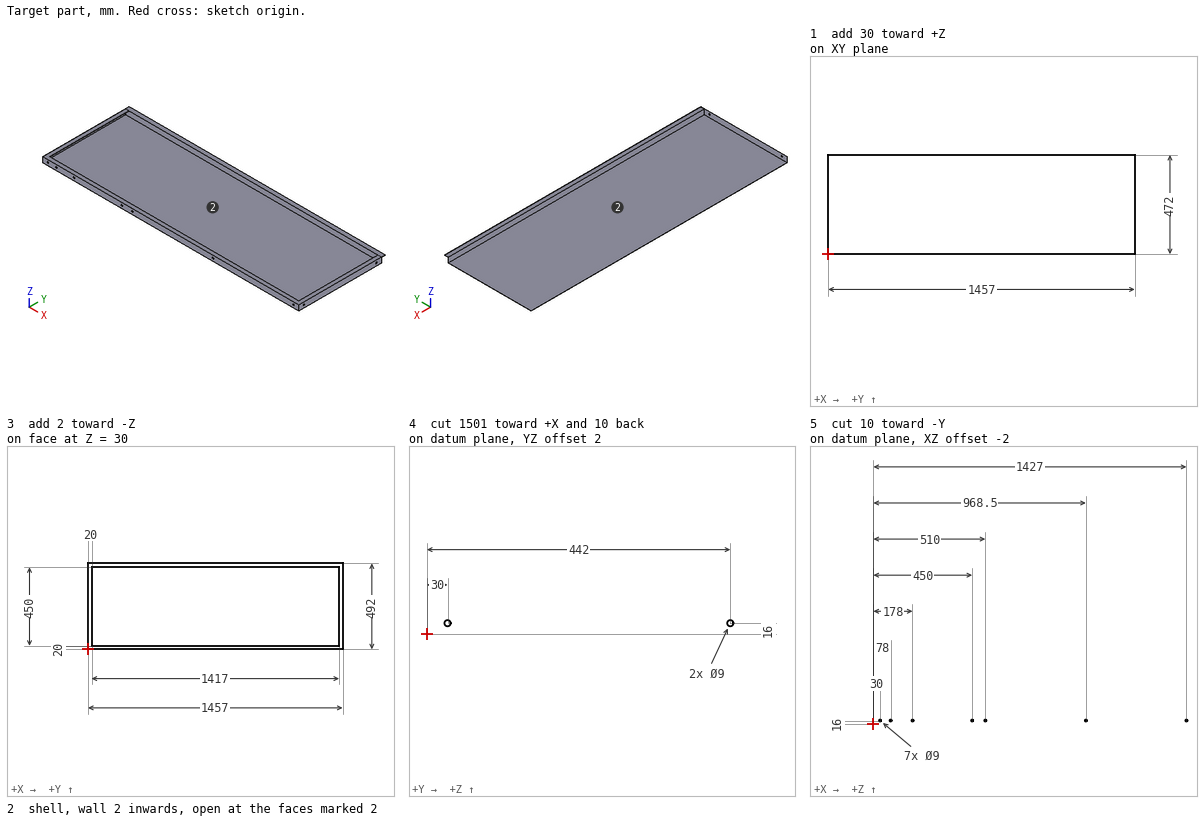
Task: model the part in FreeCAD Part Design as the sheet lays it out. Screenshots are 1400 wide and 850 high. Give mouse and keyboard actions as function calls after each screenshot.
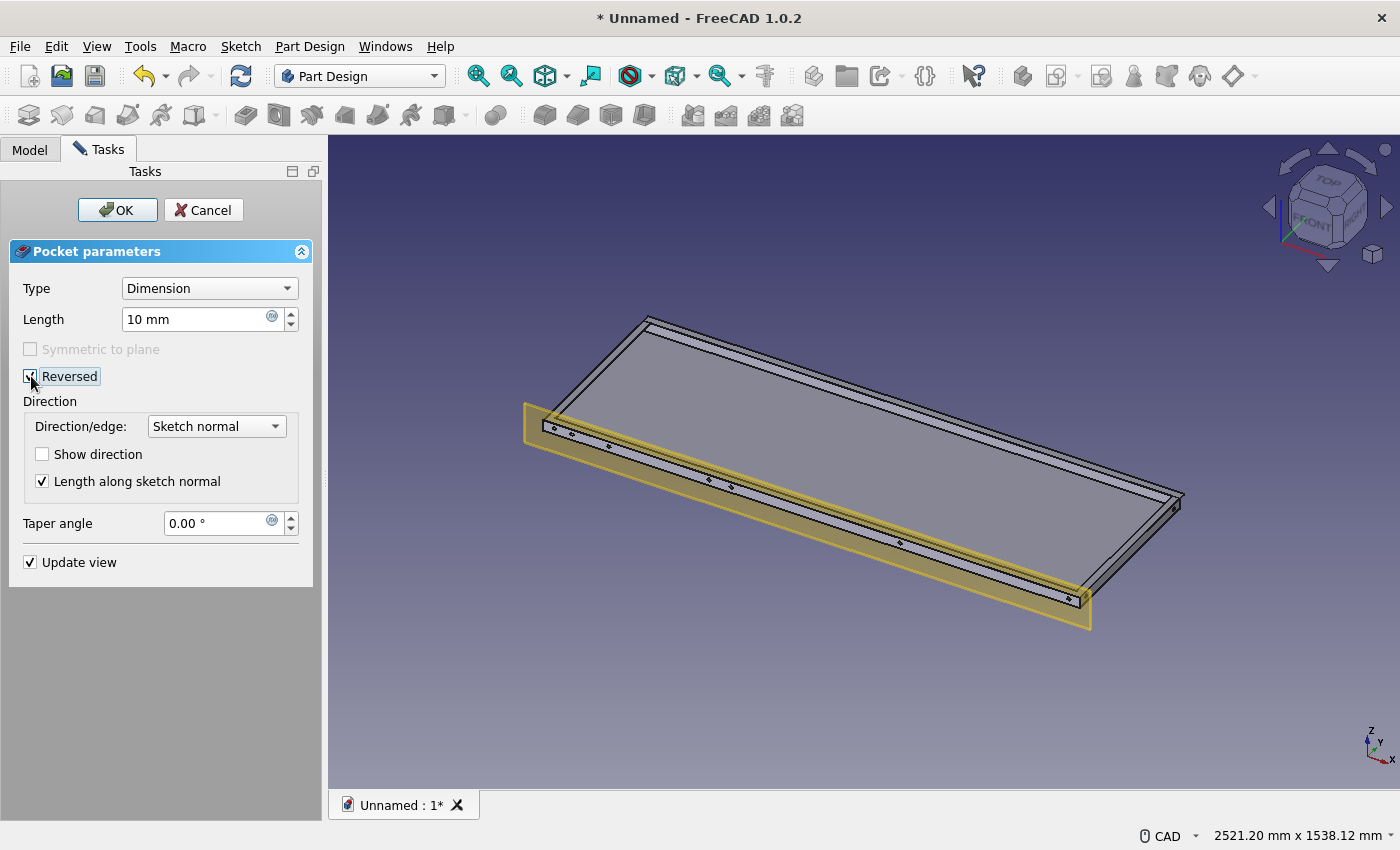
click(118, 210)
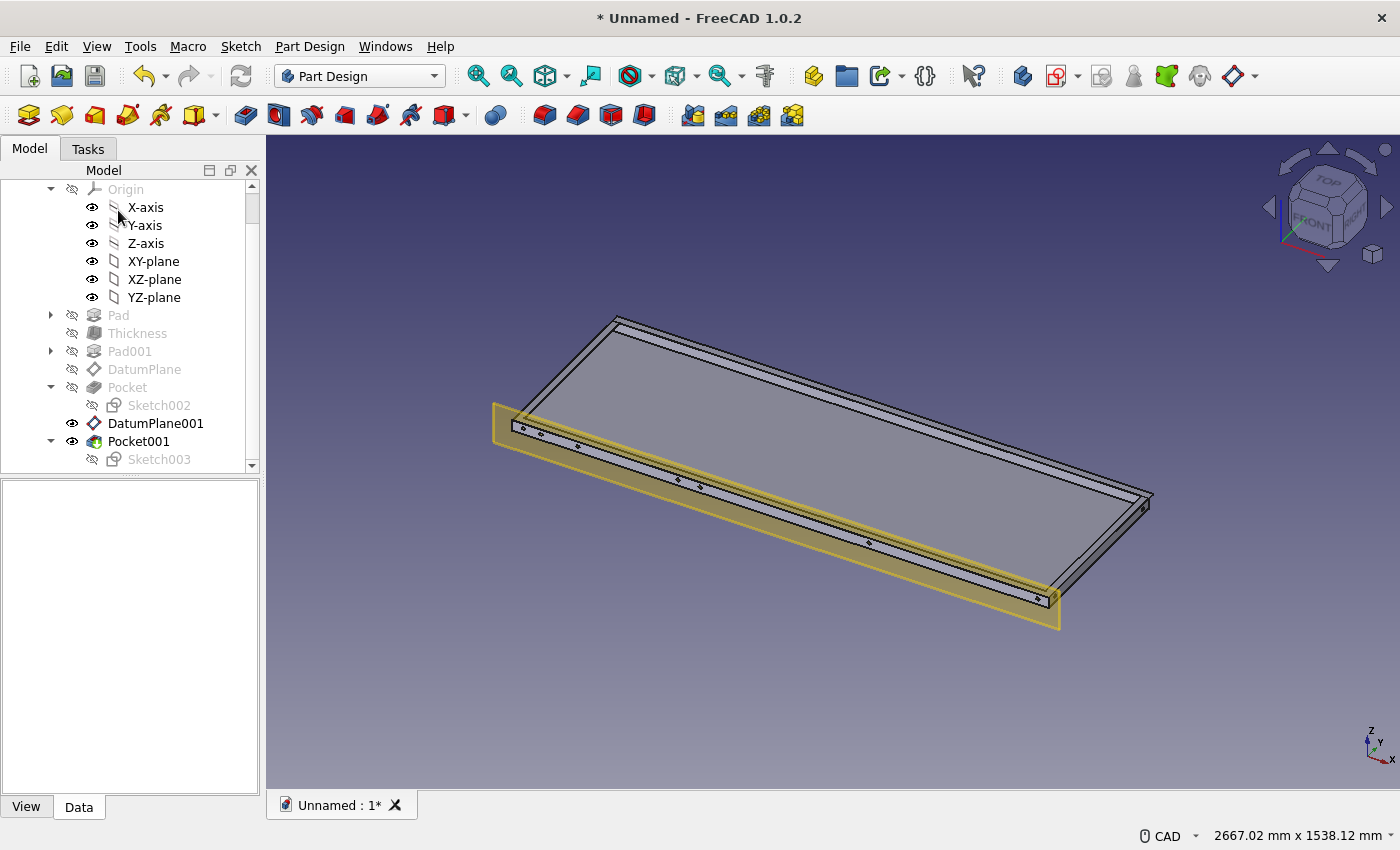
click(117, 423)
key(space)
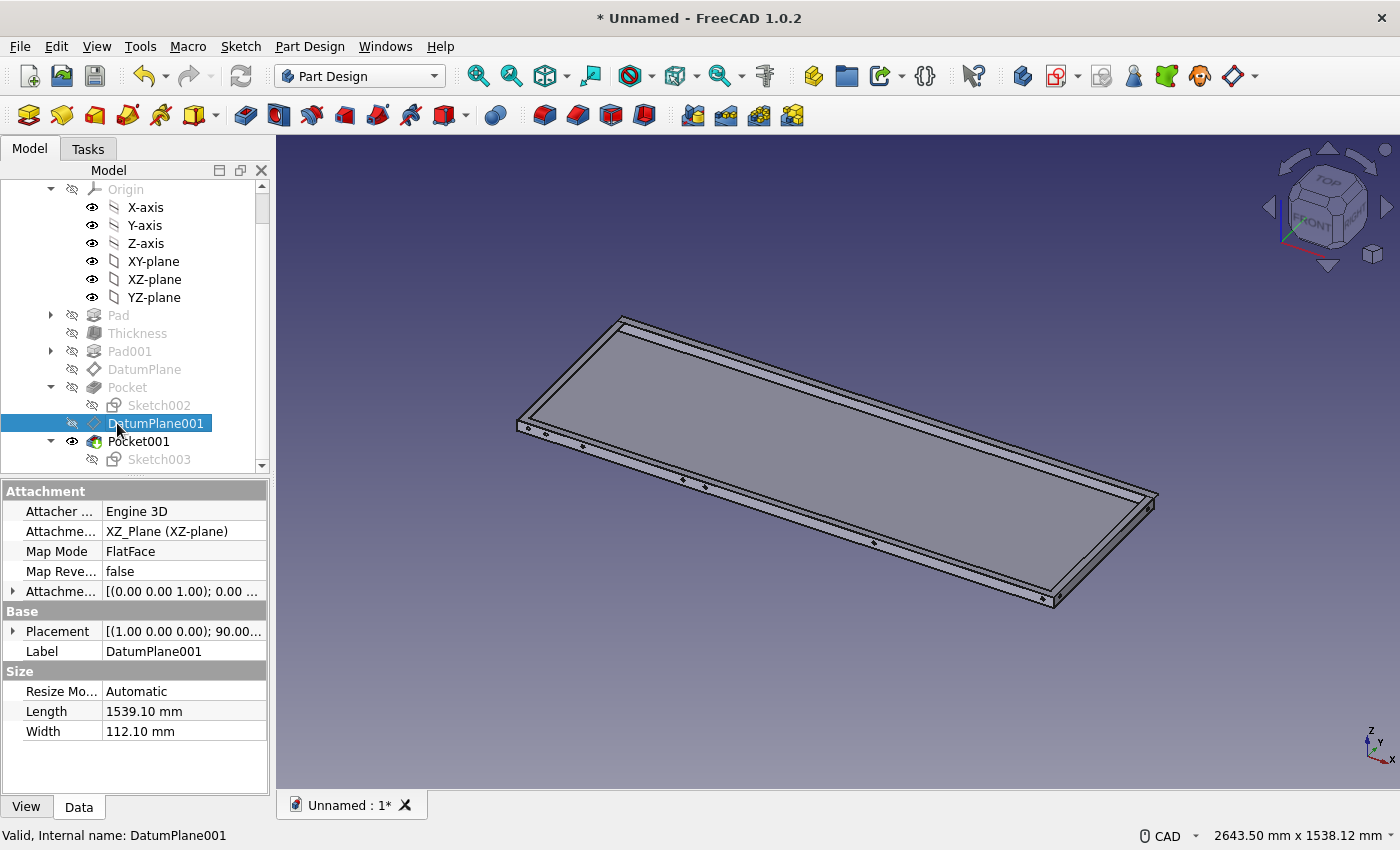
key(0)